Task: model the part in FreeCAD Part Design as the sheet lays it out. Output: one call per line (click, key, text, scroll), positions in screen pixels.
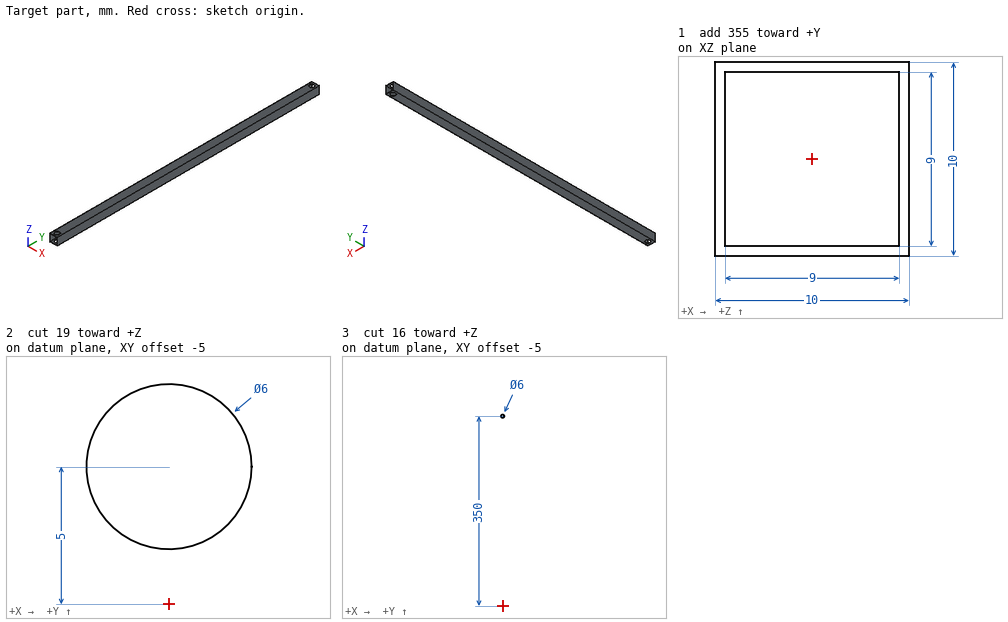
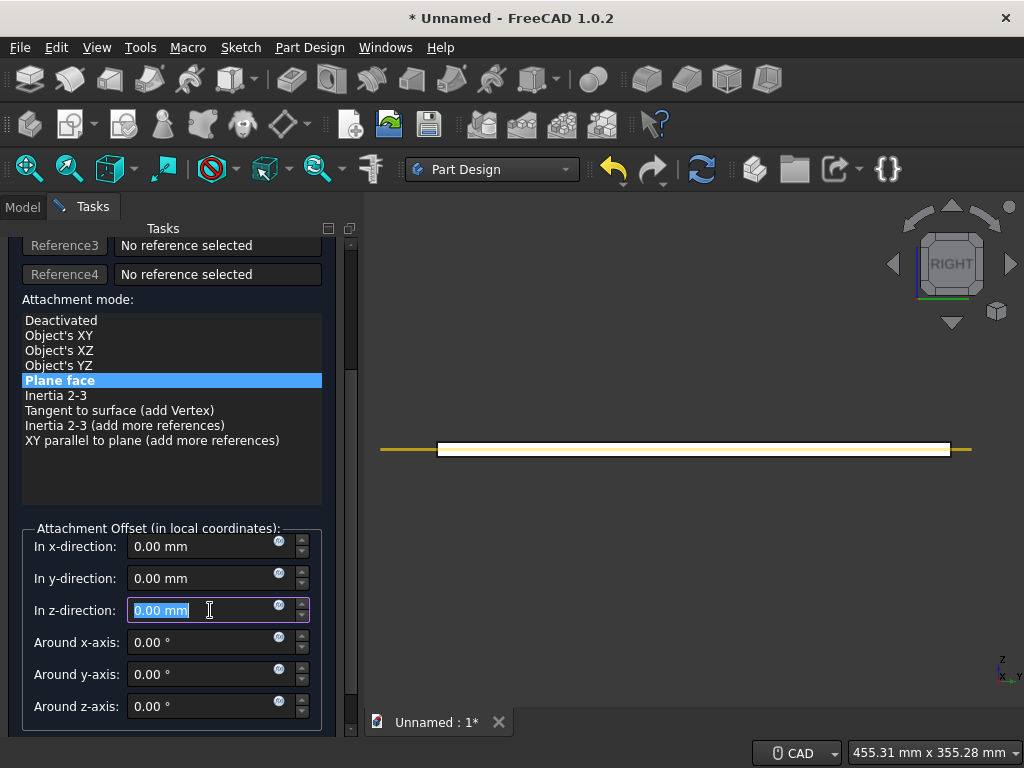
text(-5)
key(Tab)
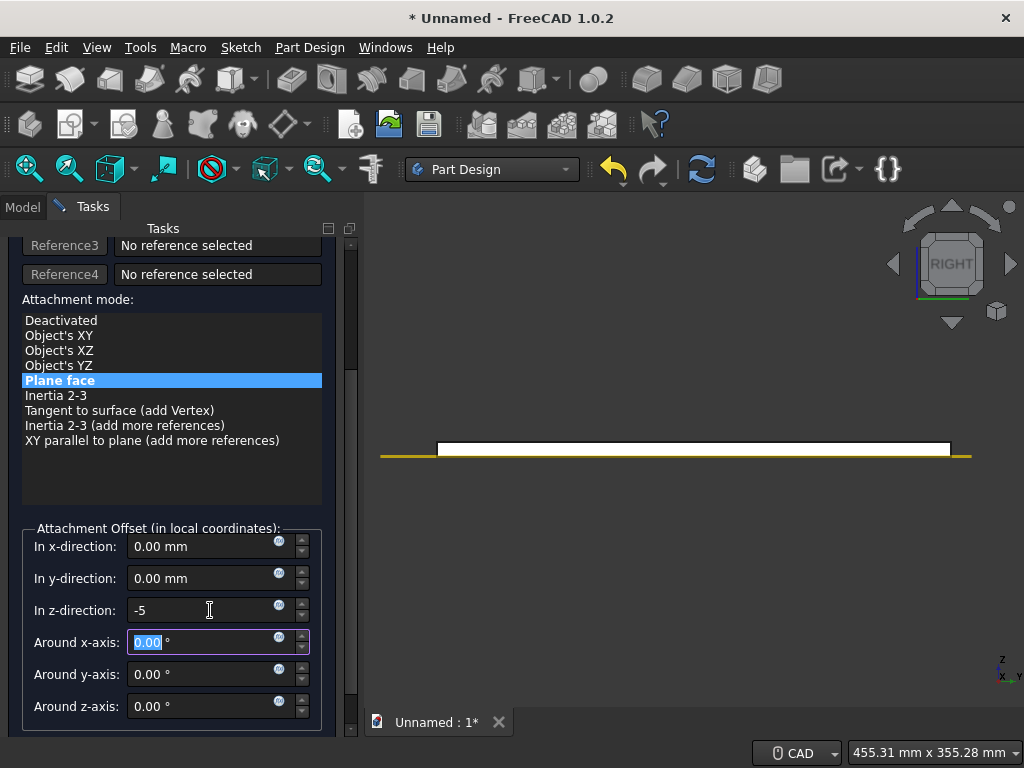
scroll(351, 487, up, 4)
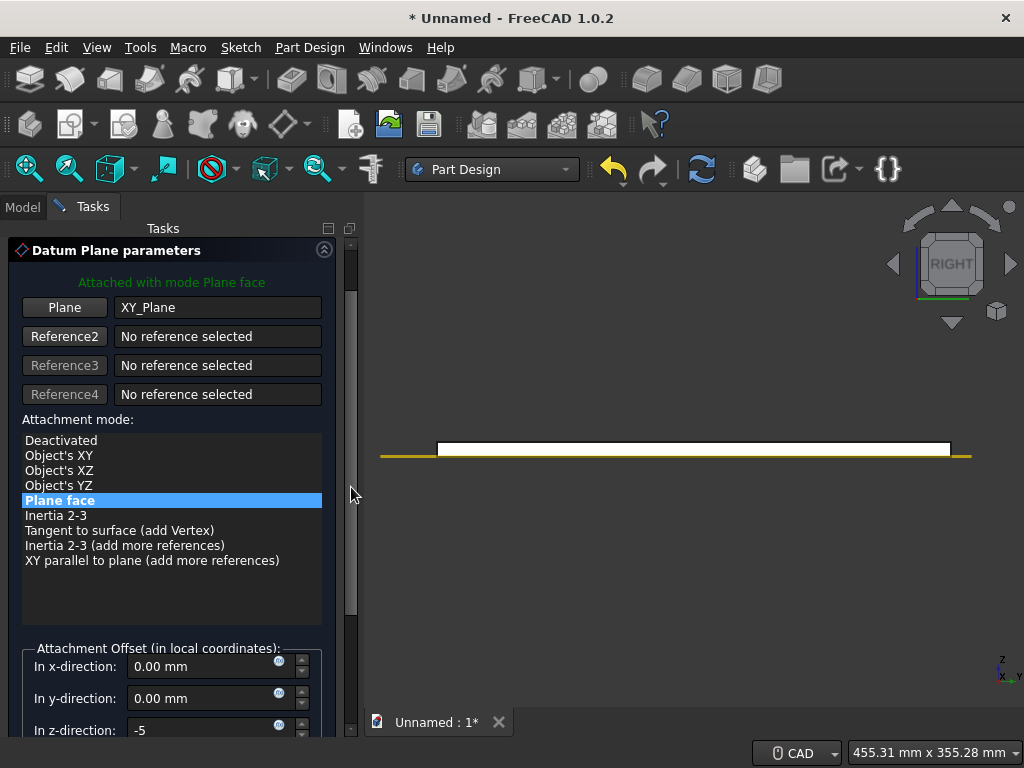
click(124, 267)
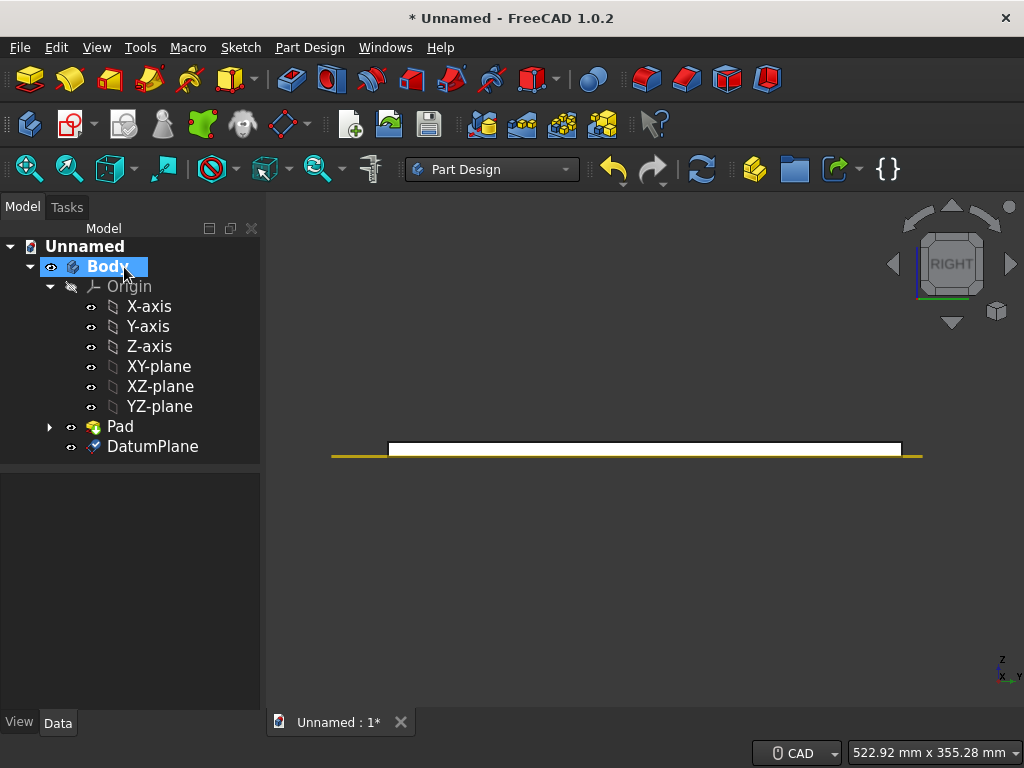
click(116, 447)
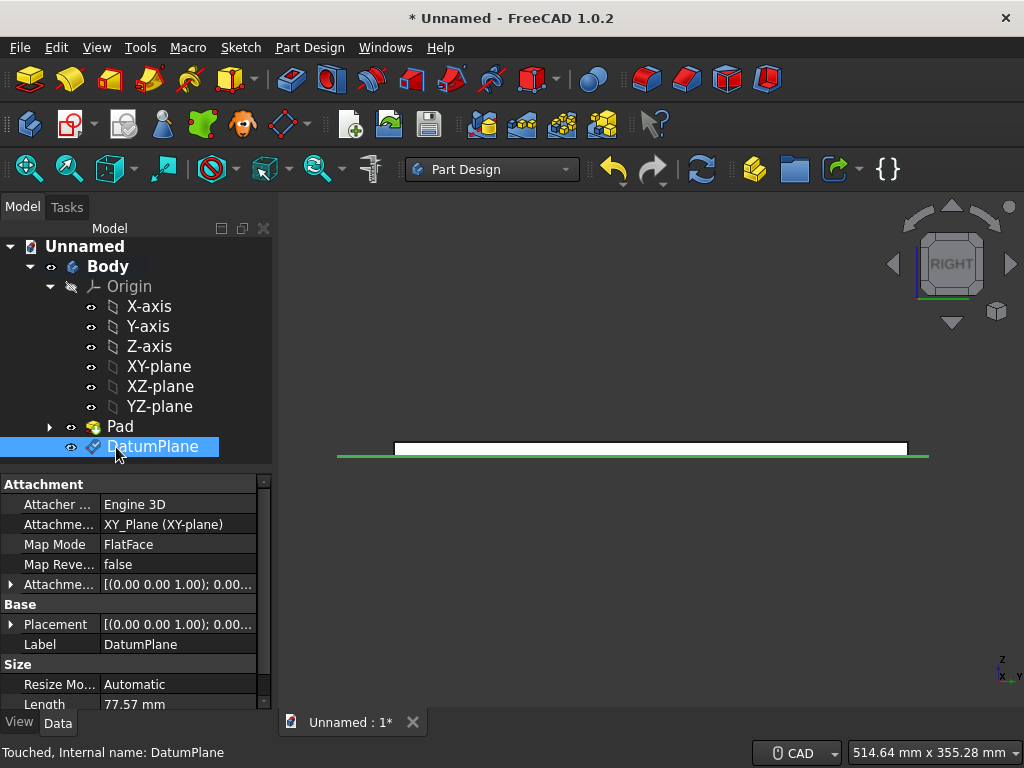
click(70, 124)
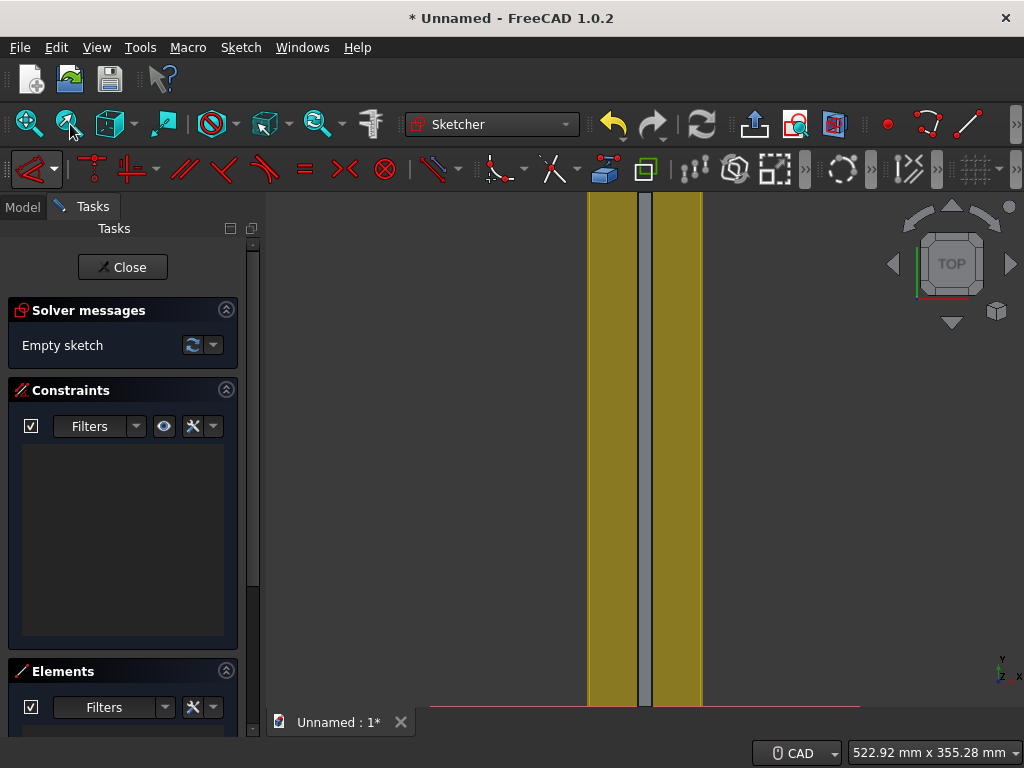
click(836, 124)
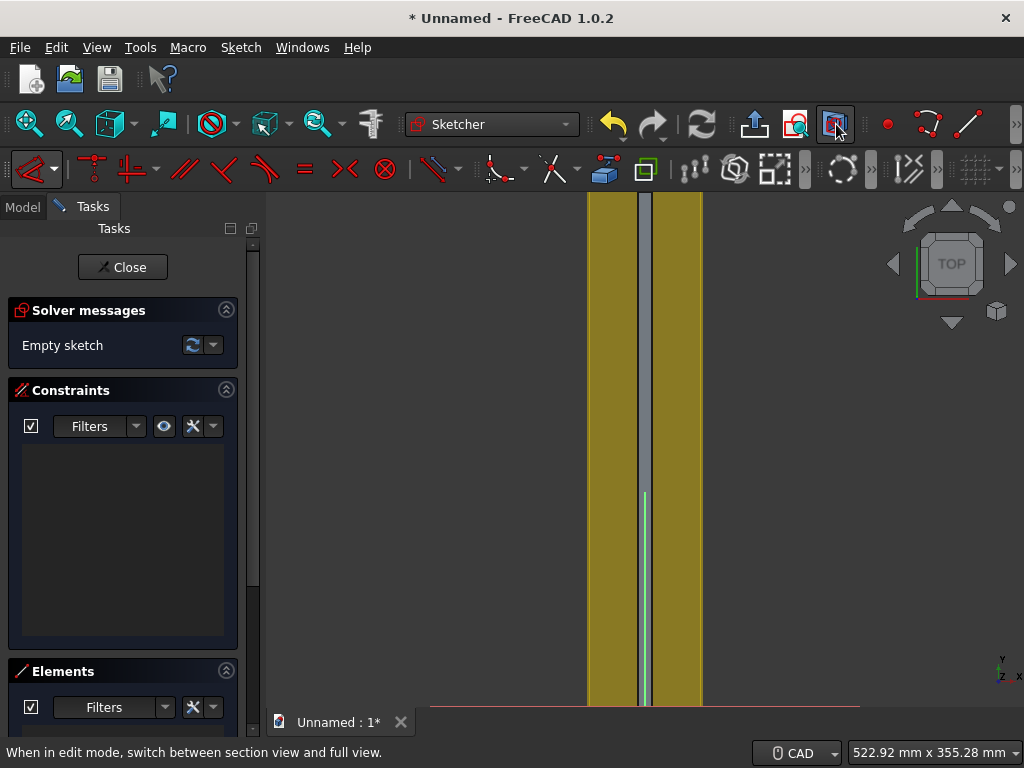
scroll(576, 450, down, 5)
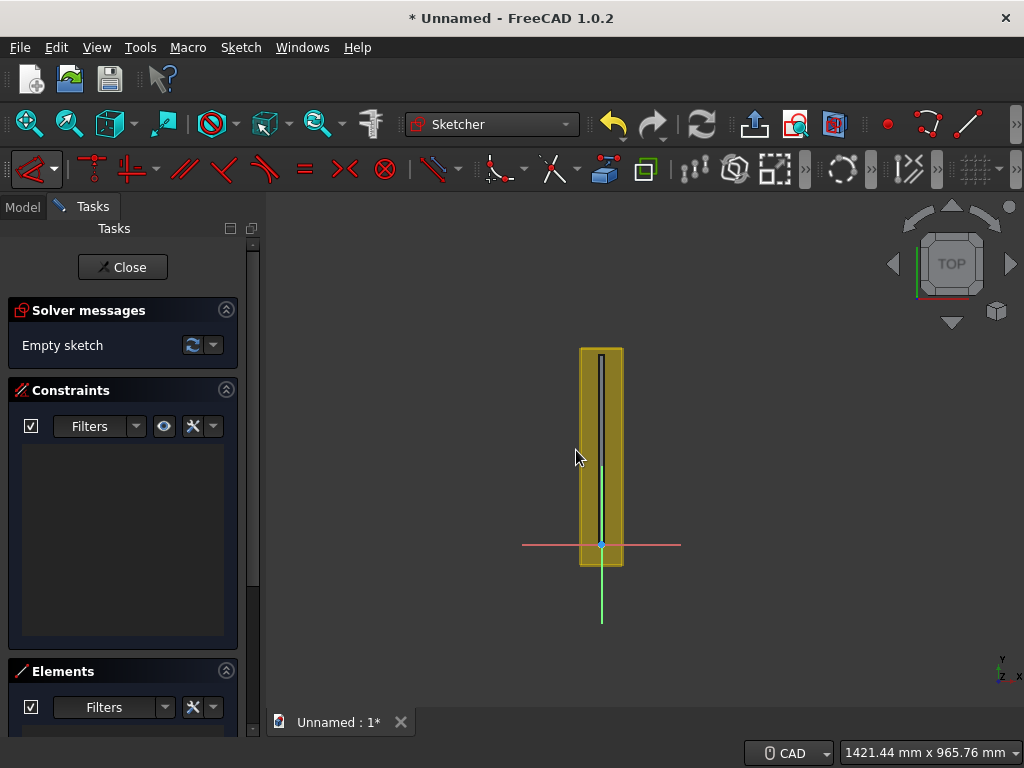
scroll(603, 548, up, 15)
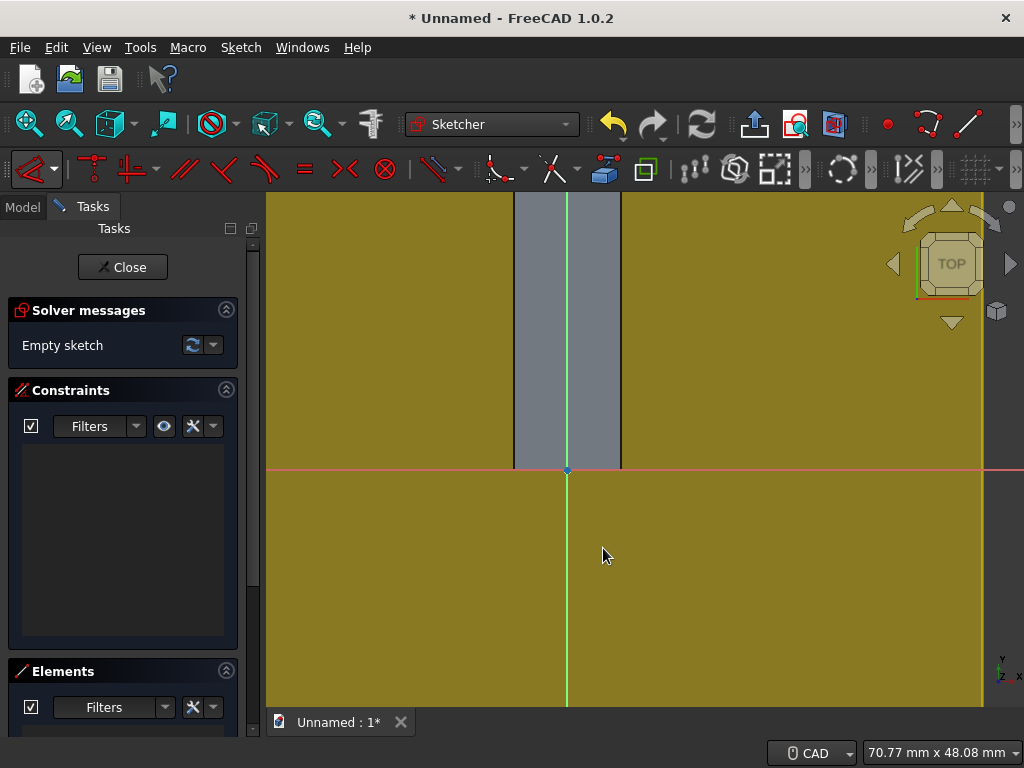
scroll(564, 420, up, 7)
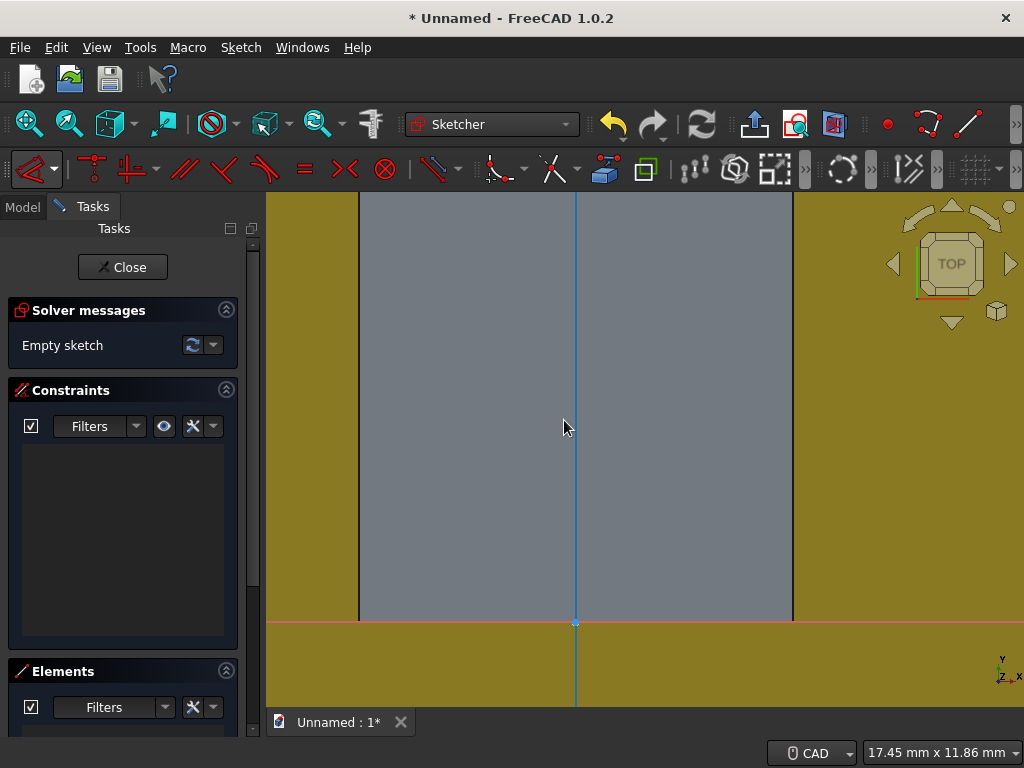
key(g)
key(c)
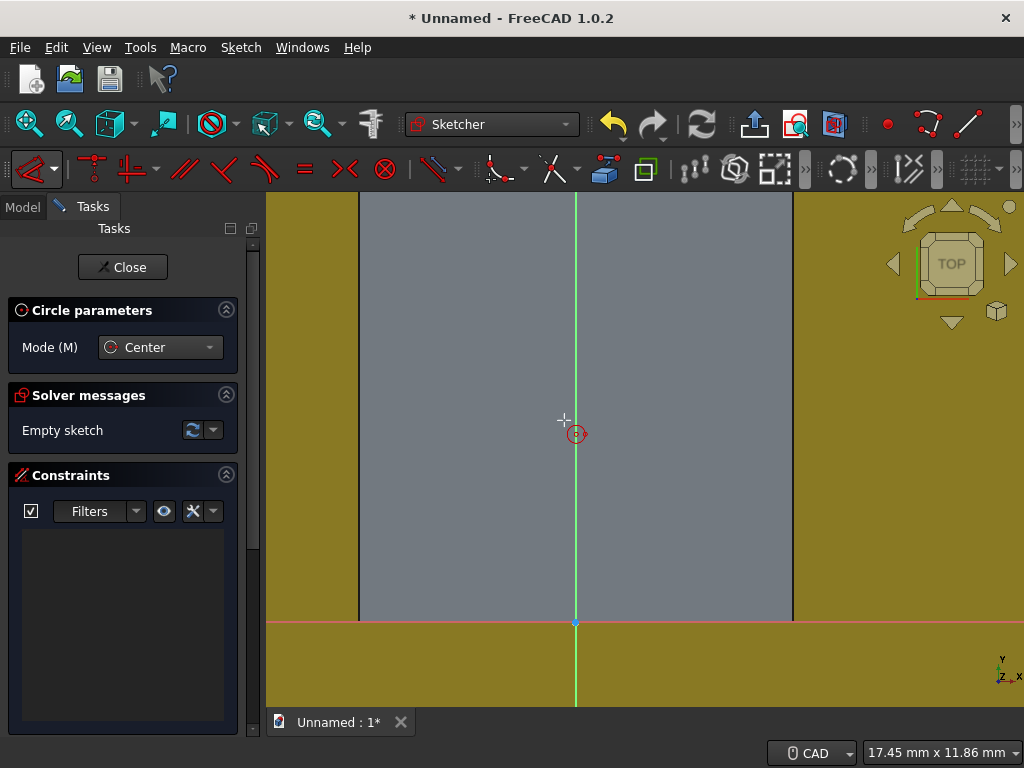
click(576, 405)
move(668, 313)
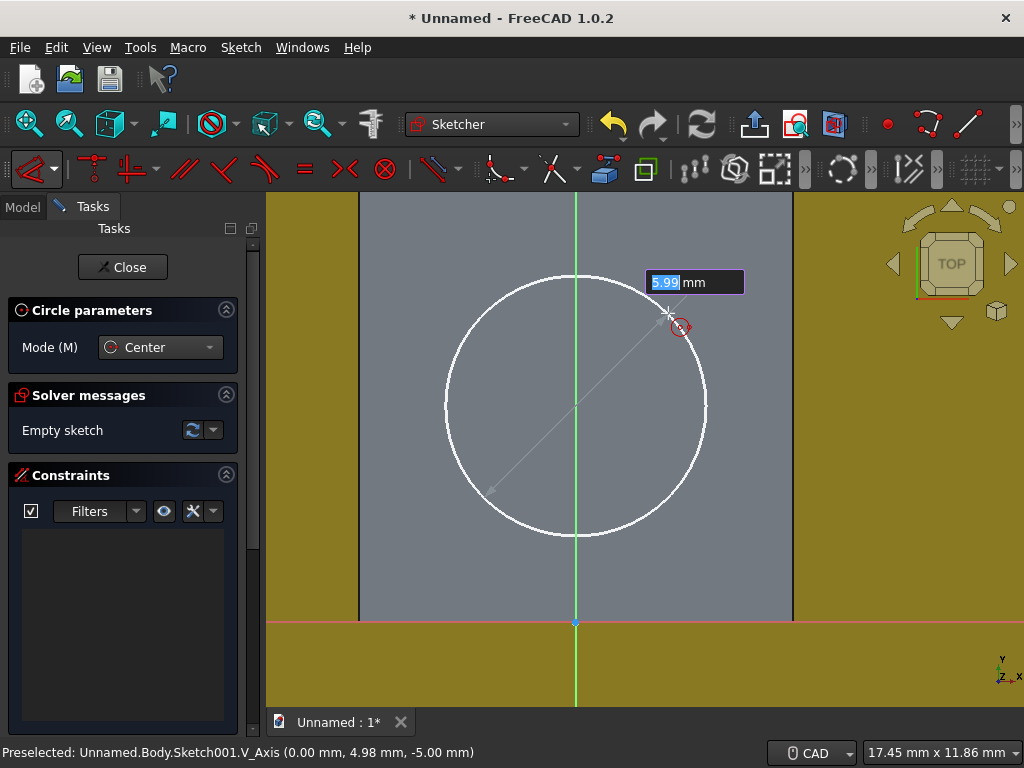
text(6)
key(Return)
key(Escape)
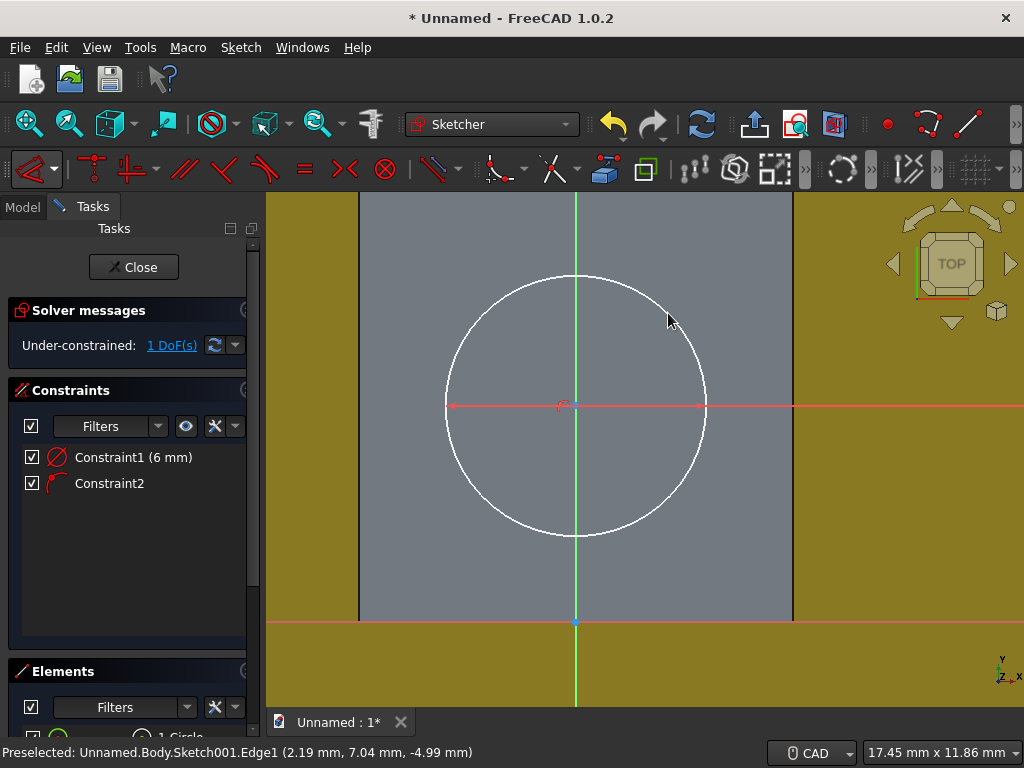
click(30, 170)